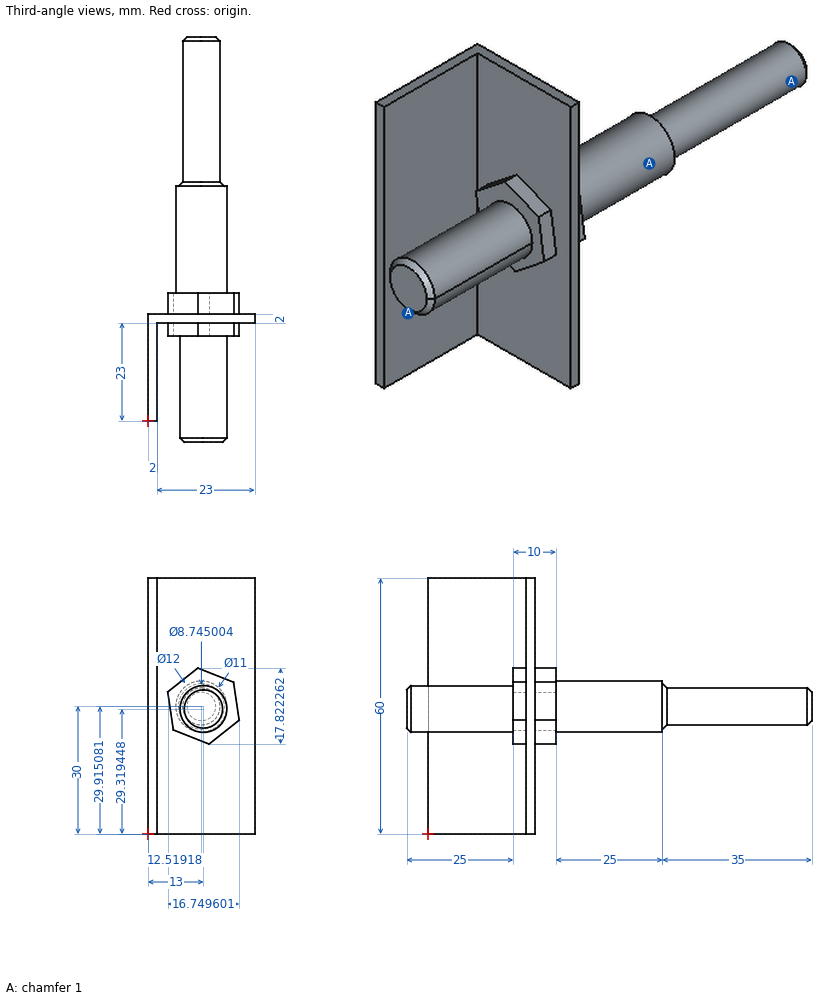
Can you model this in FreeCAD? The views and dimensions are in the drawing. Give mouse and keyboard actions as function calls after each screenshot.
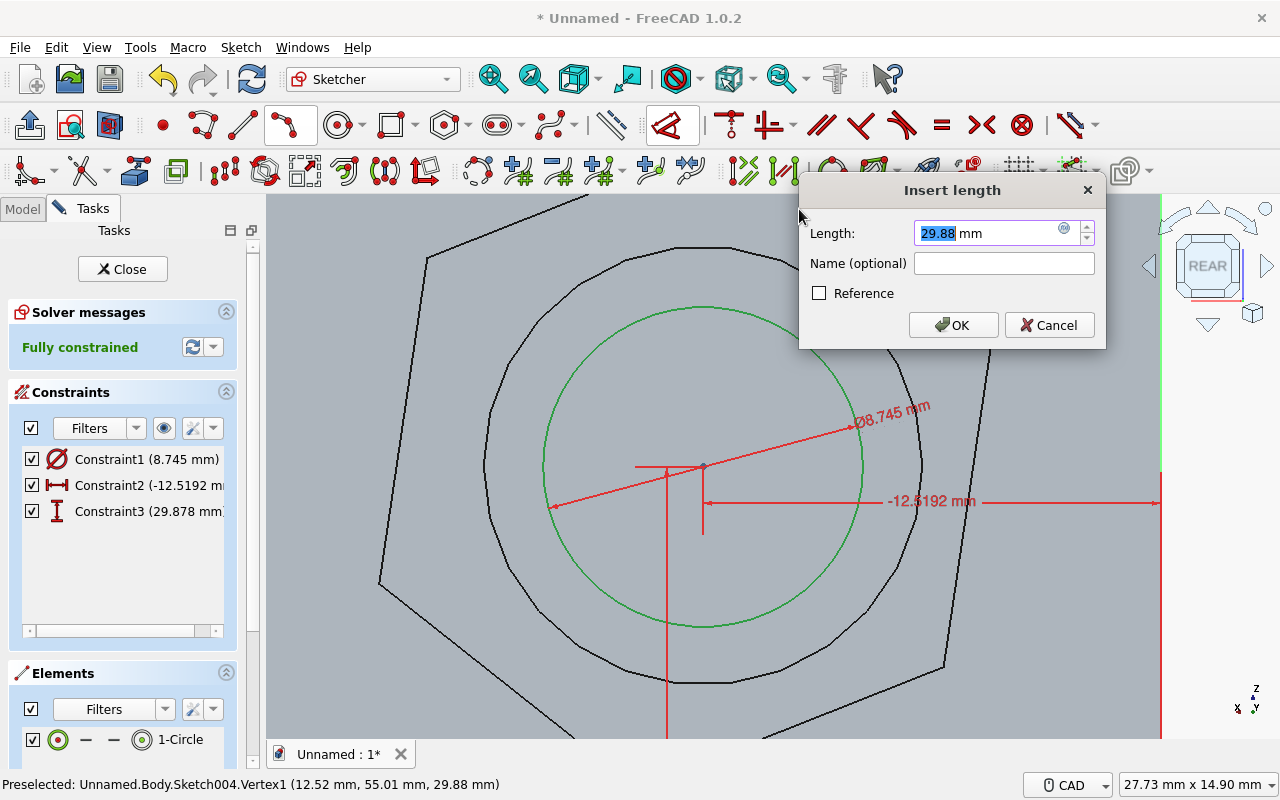
text(29.915081)
key(Return)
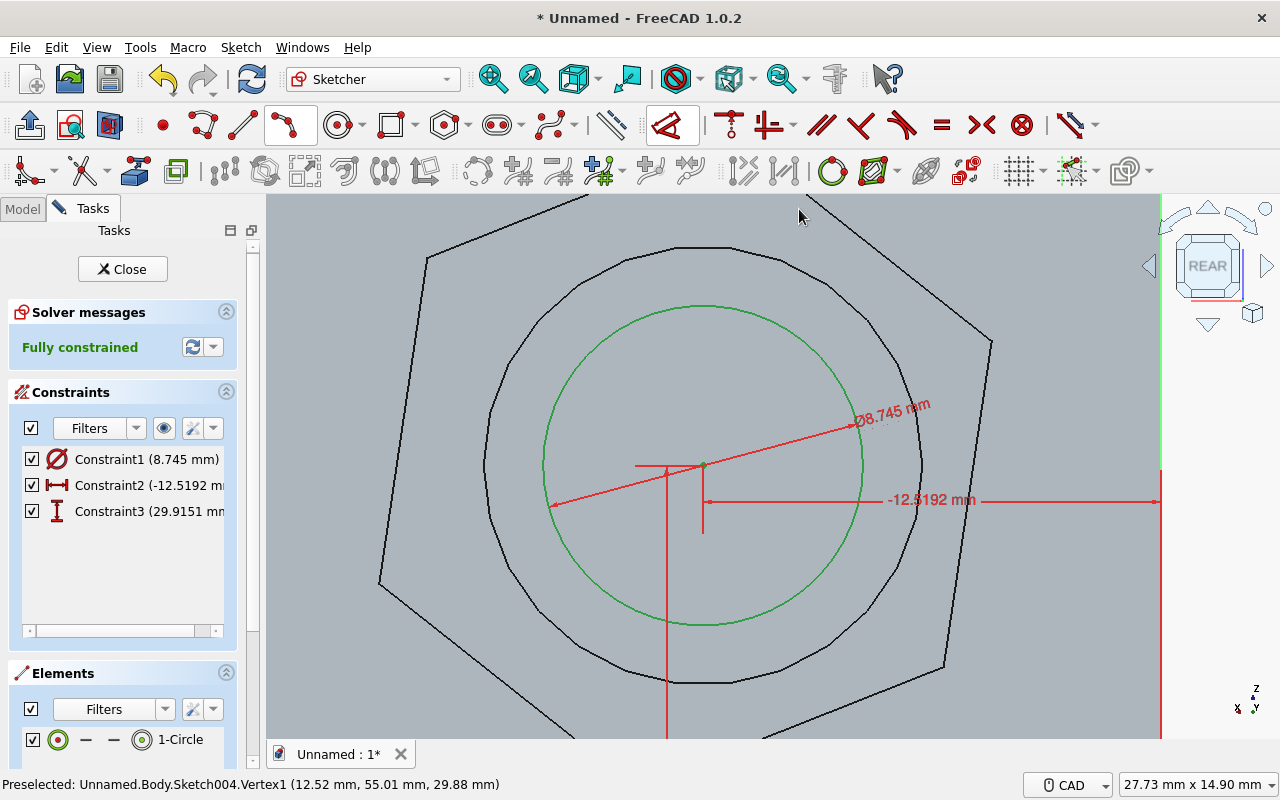
click(123, 269)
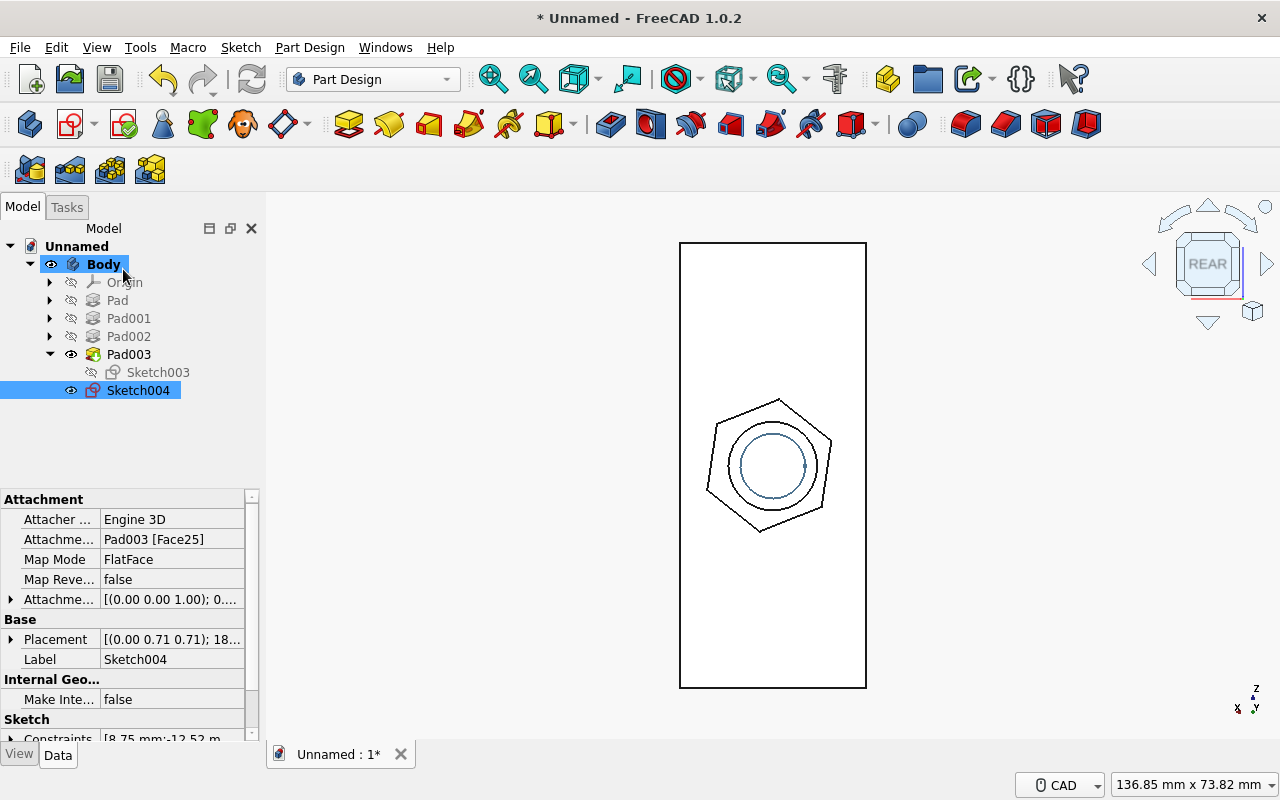
click(350, 124)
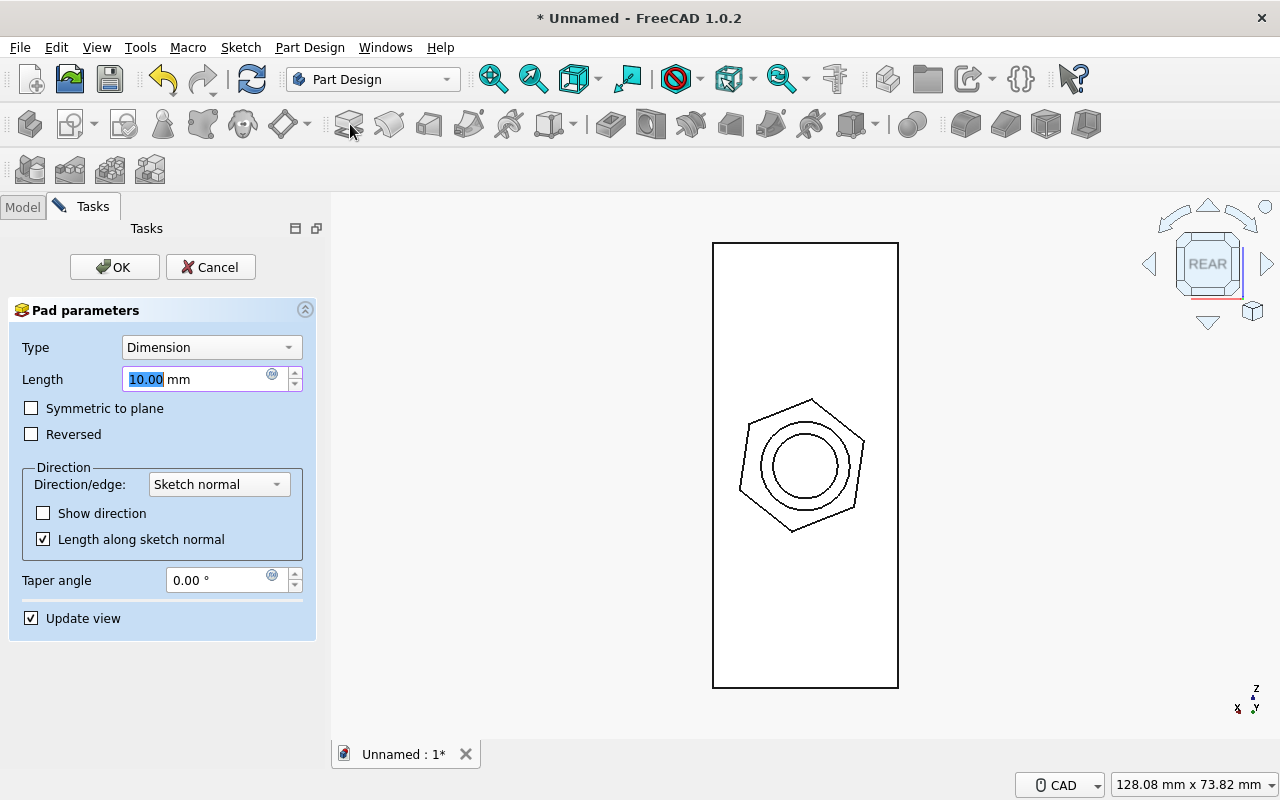
text(35)
key(Tab)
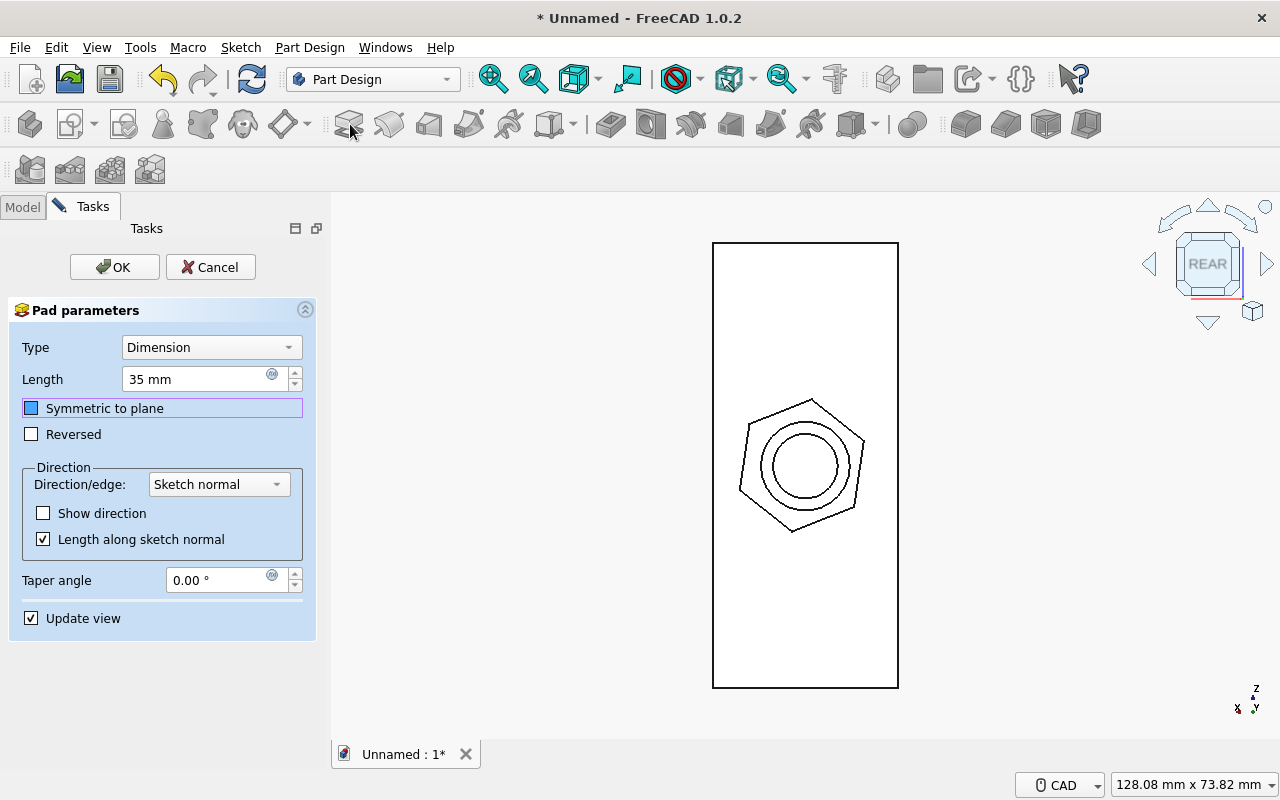
click(115, 267)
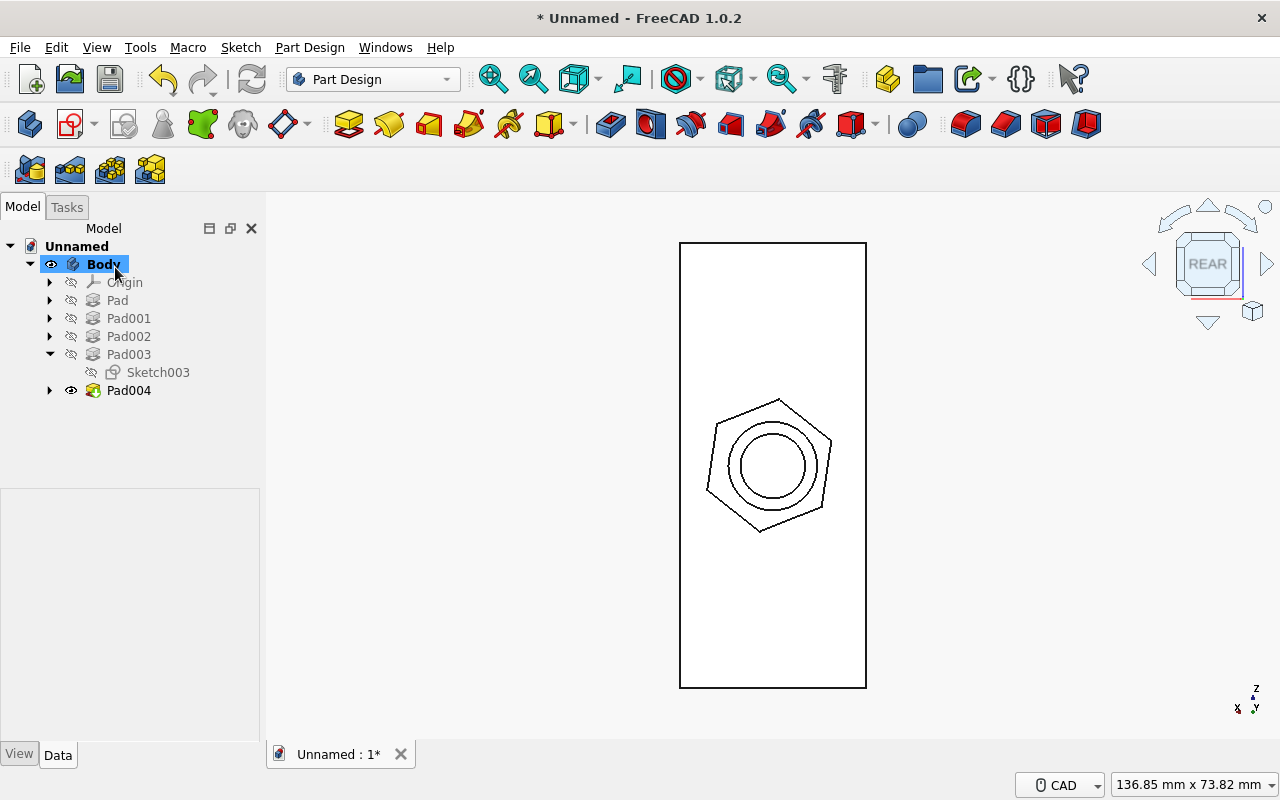
click(747, 446)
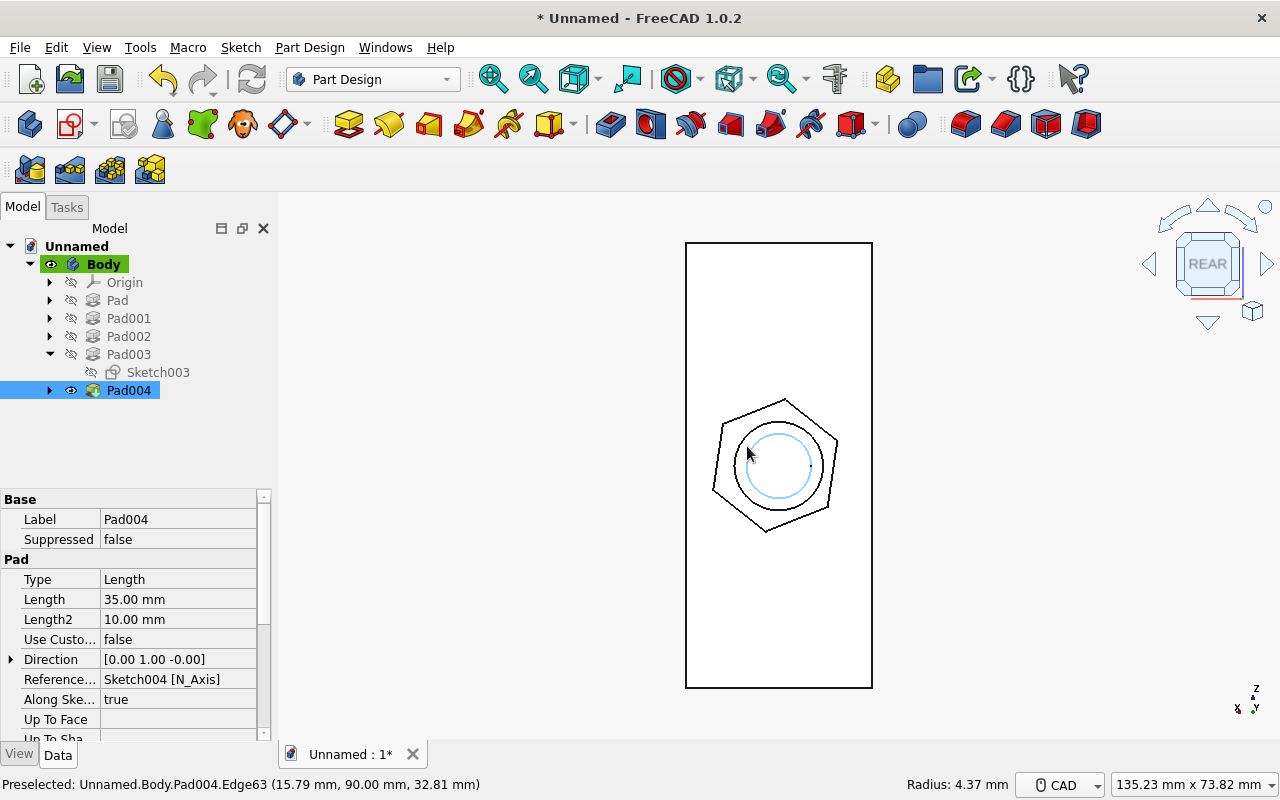
key(0)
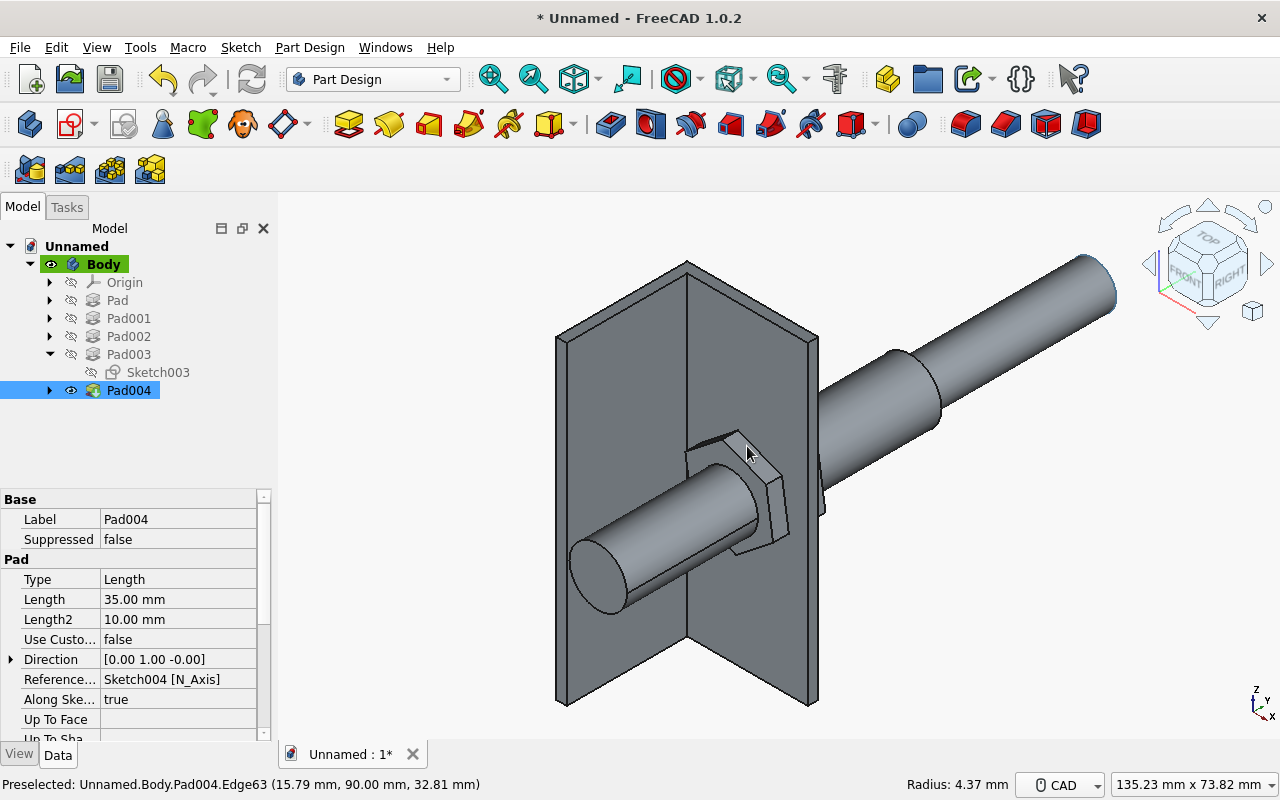
key(v)
key(f)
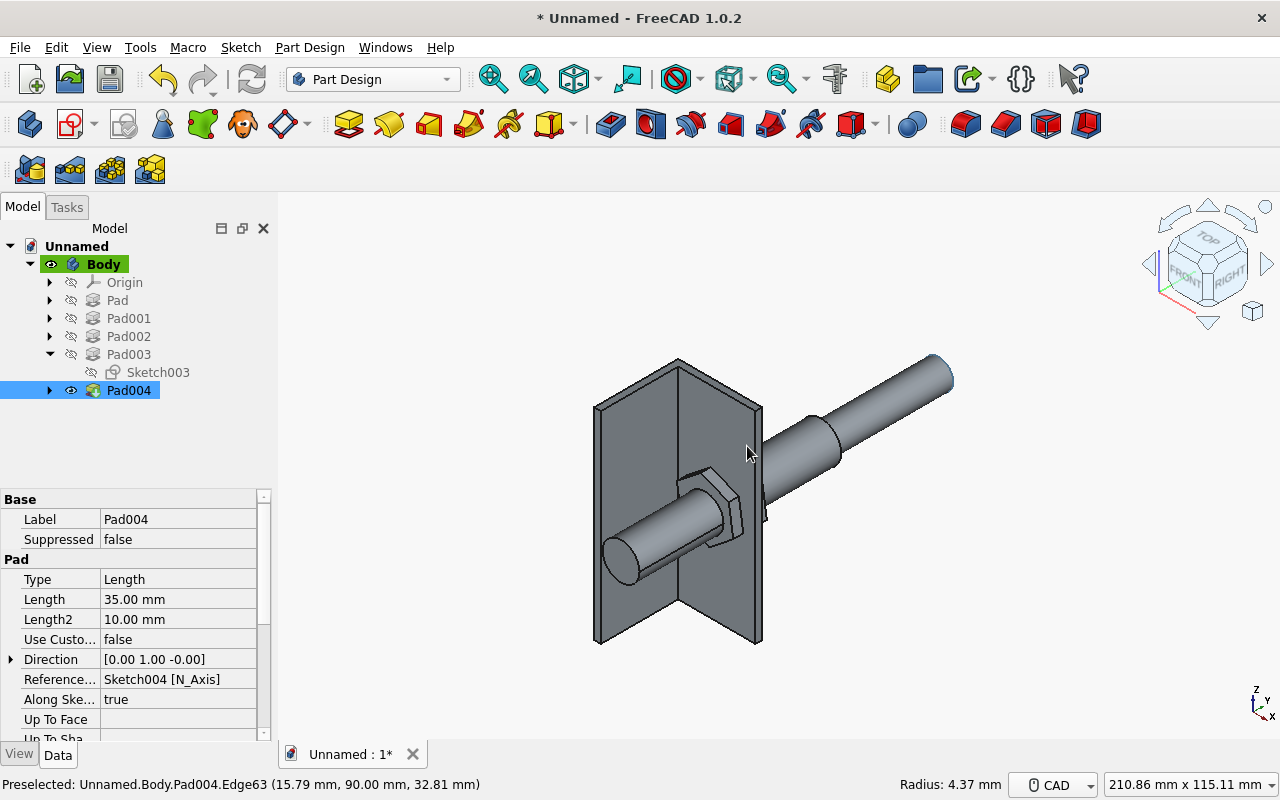
click(606, 539, ctrl)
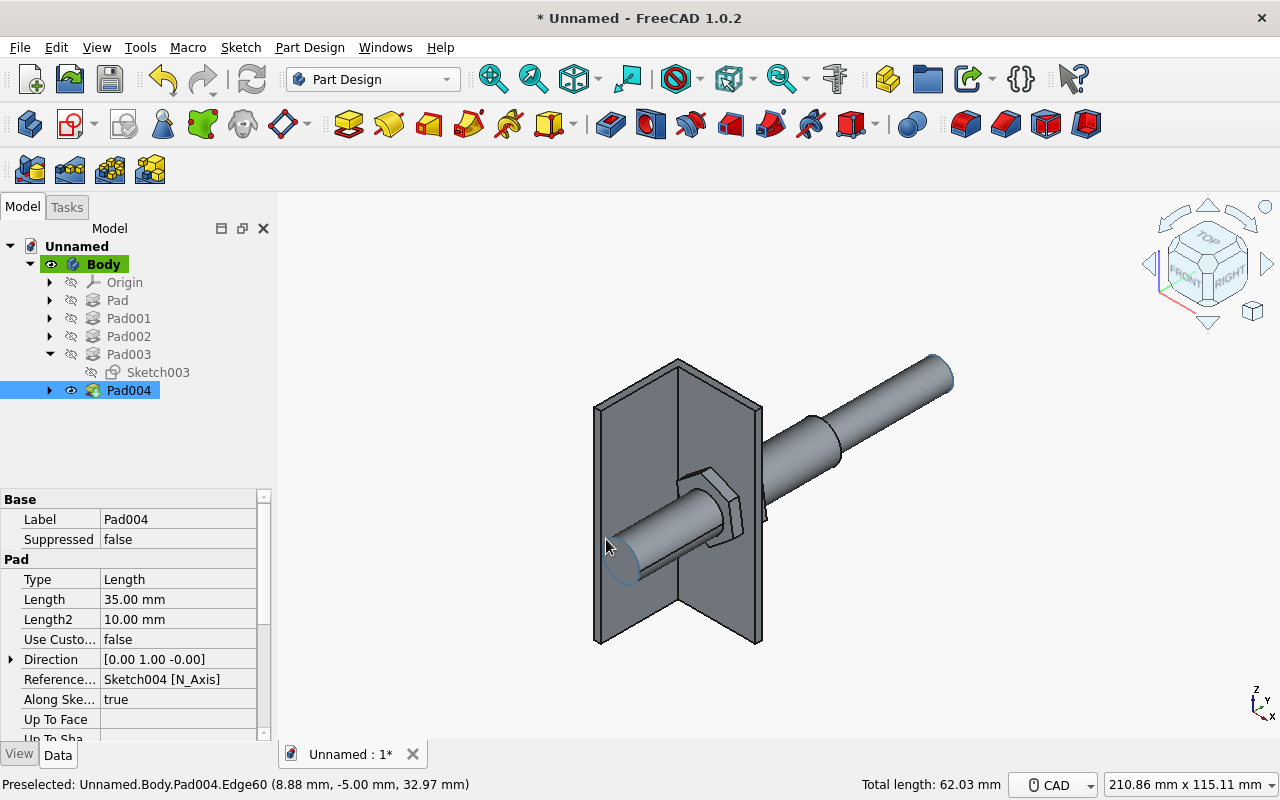
key(2)